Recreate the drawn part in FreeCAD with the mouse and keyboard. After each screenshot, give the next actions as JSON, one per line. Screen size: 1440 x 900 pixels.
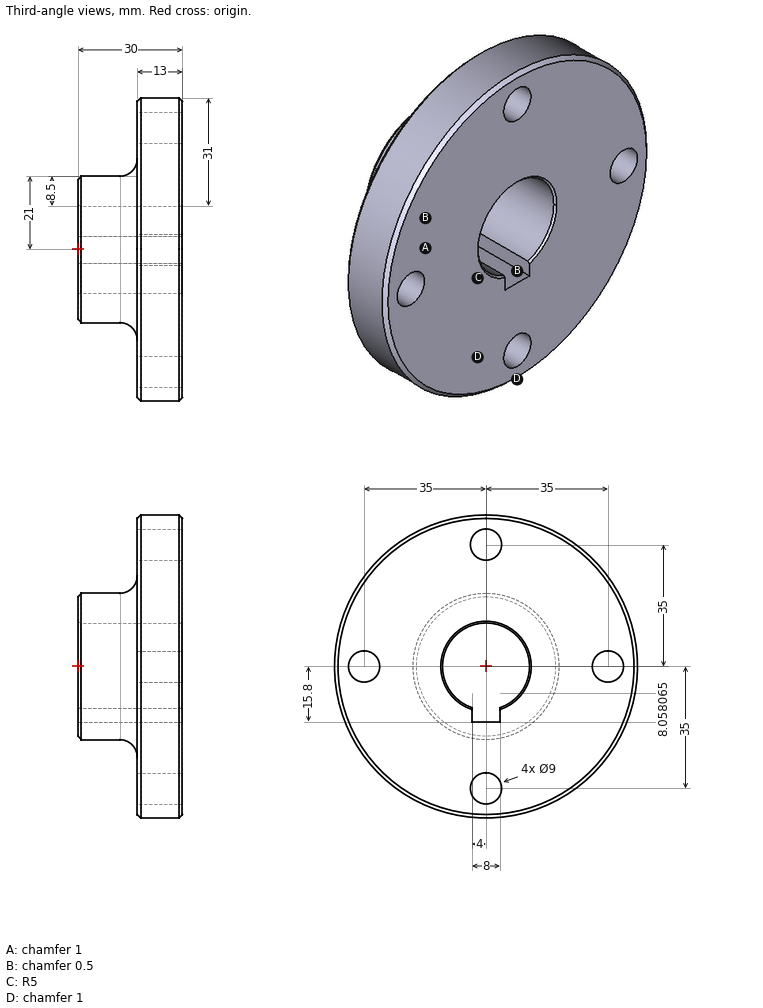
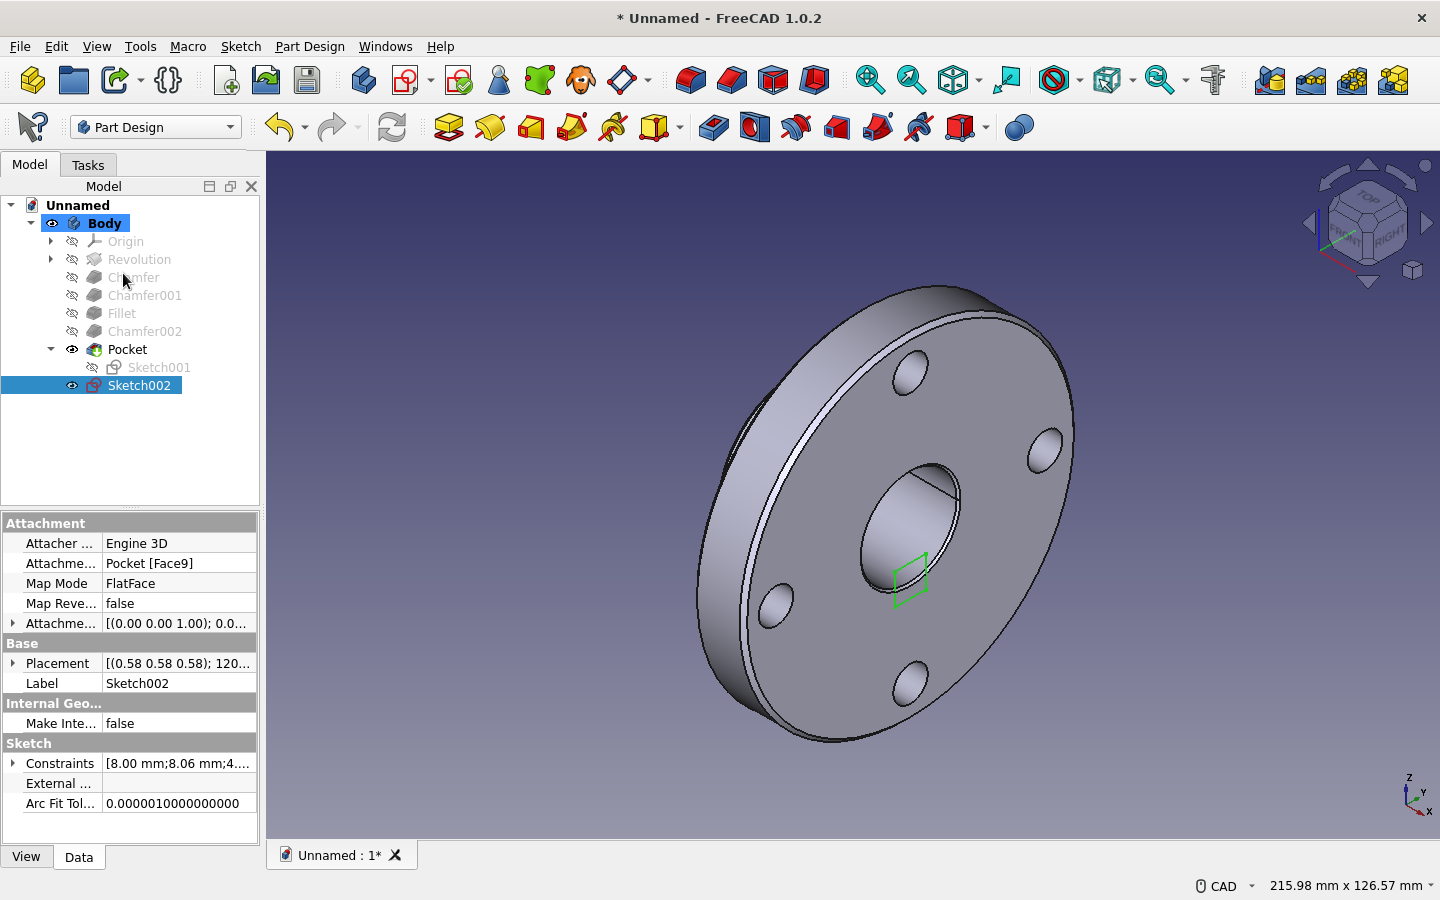
{"action": "left_click", "coordinate": [714, 128]}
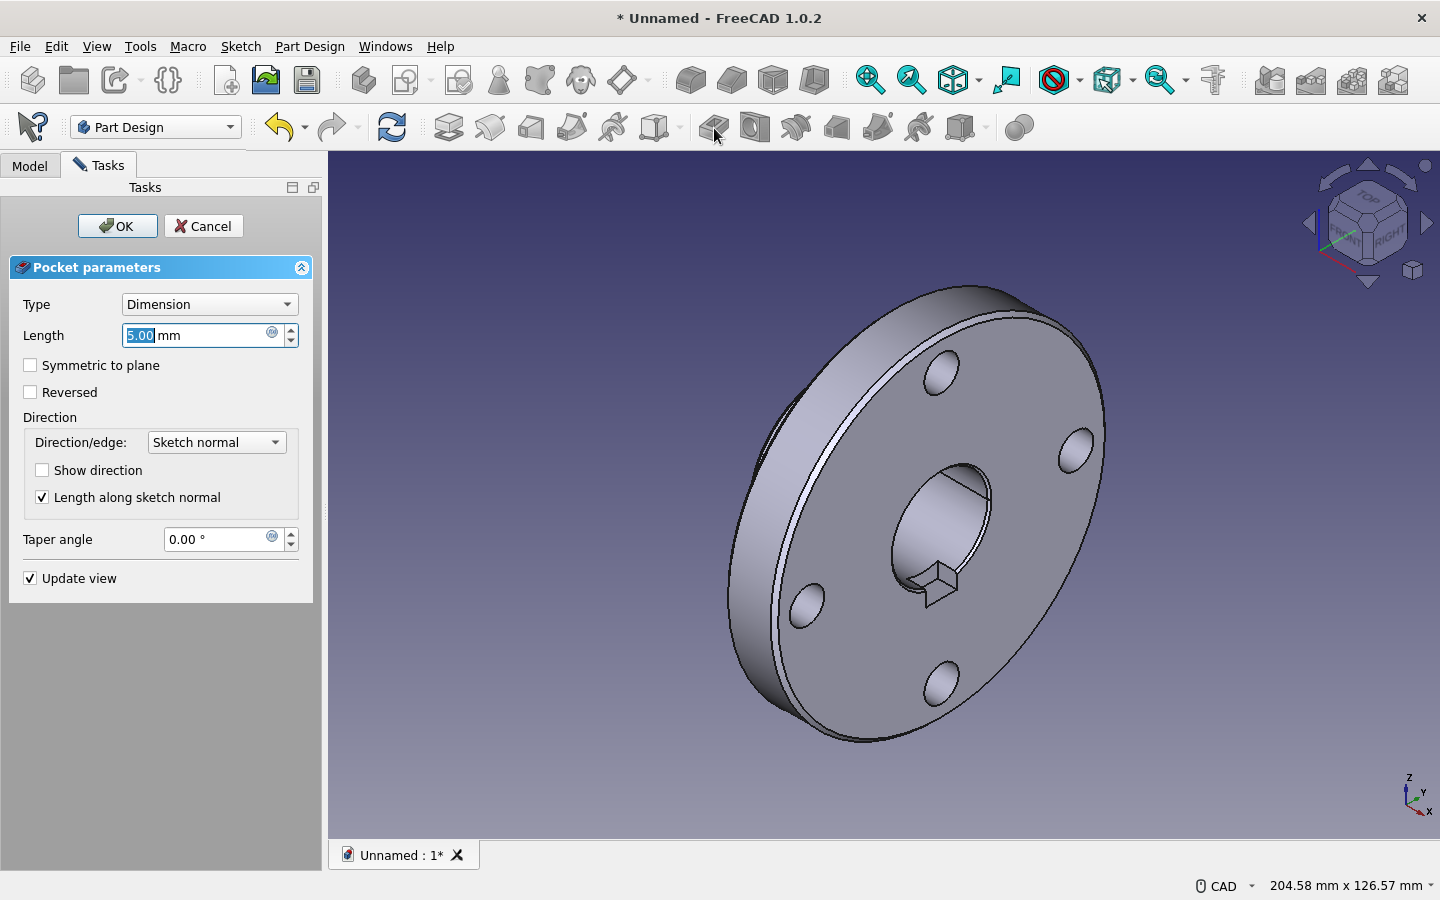
{"action": "left_click", "coordinate": [210, 304]}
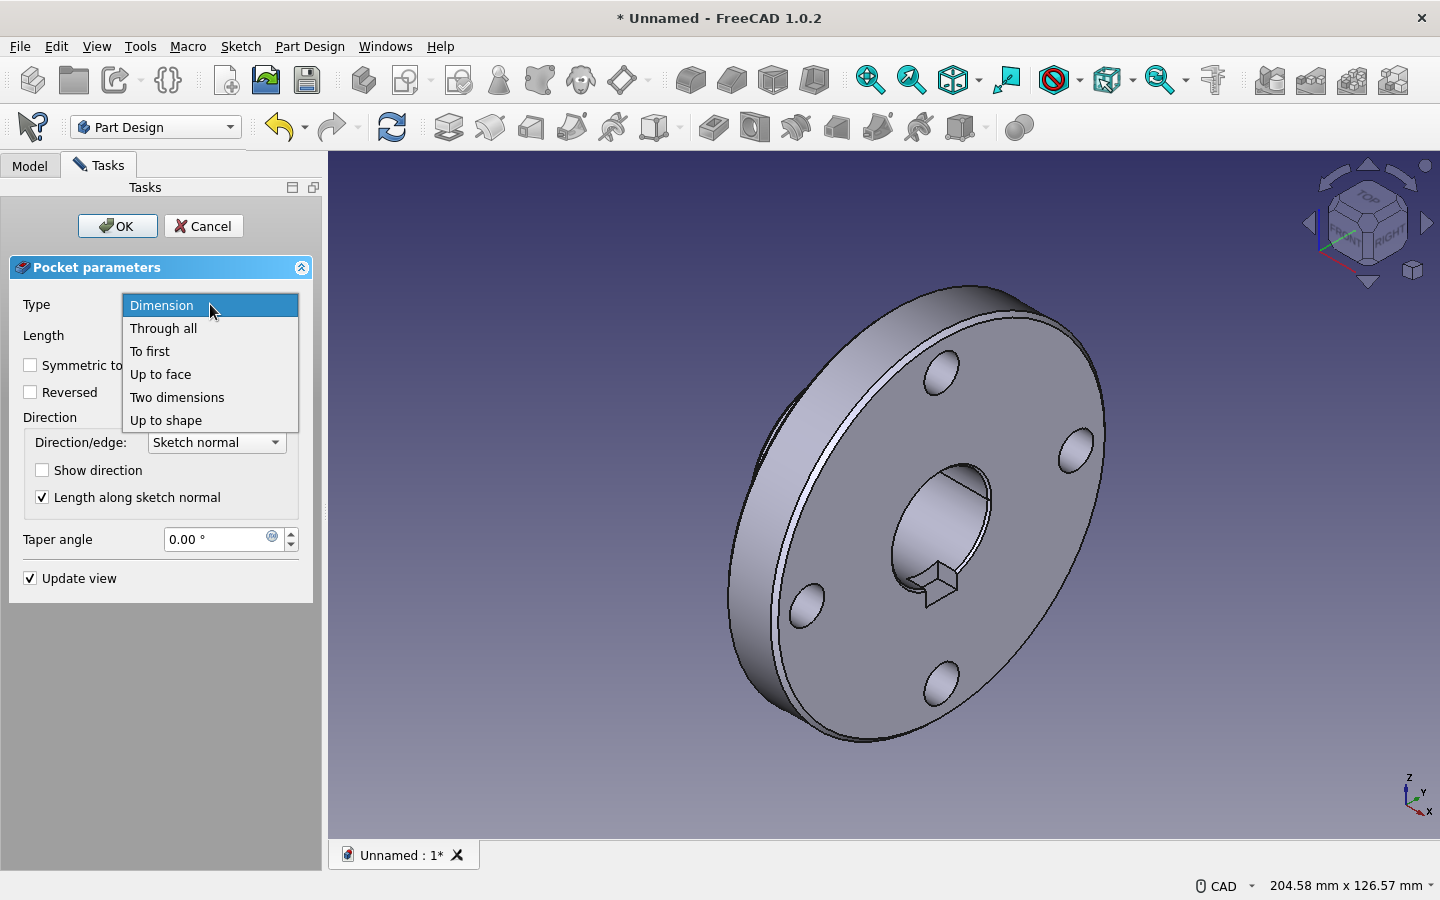
{"action": "left_click", "coordinate": [208, 328]}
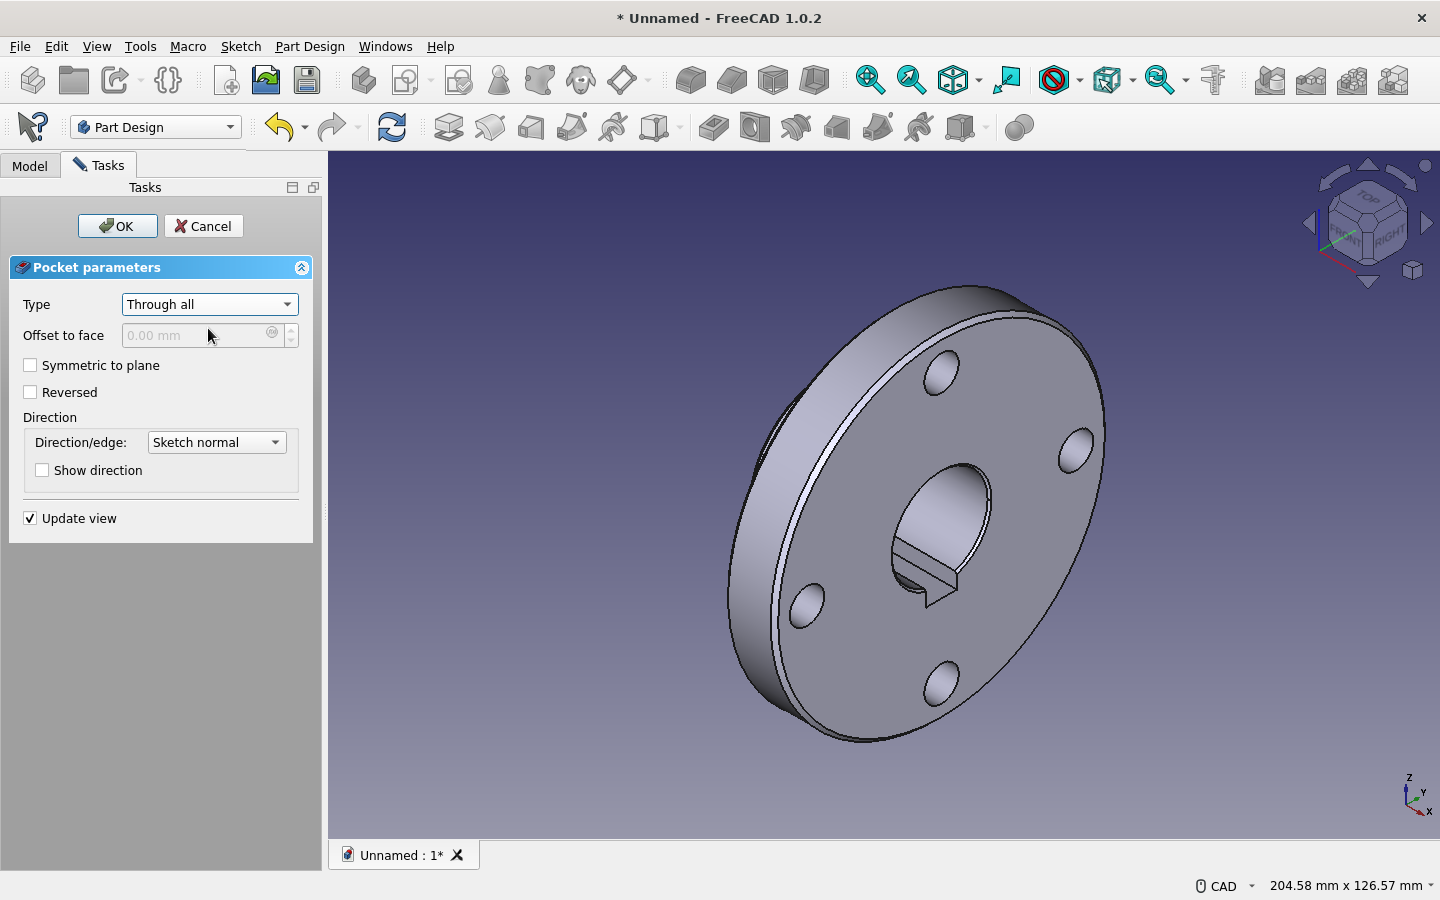
{"action": "left_click", "coordinate": [118, 226]}